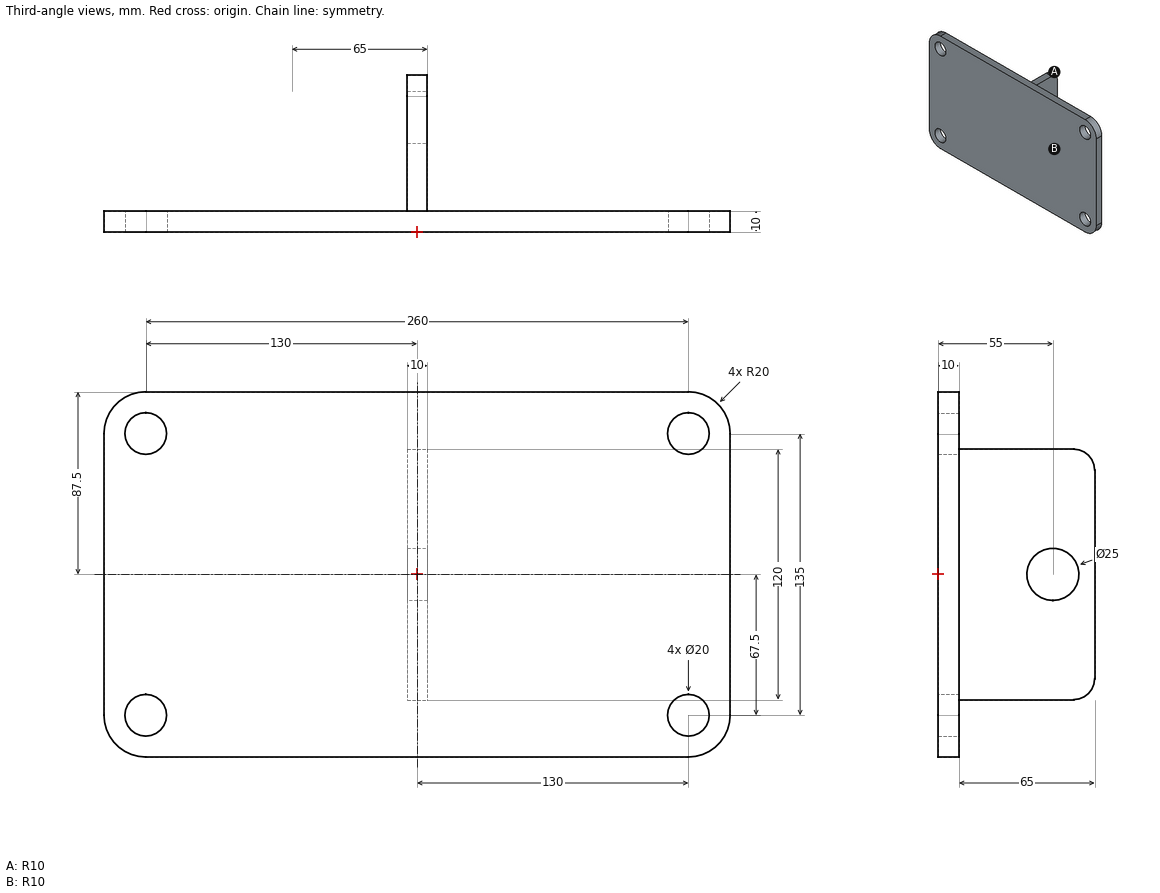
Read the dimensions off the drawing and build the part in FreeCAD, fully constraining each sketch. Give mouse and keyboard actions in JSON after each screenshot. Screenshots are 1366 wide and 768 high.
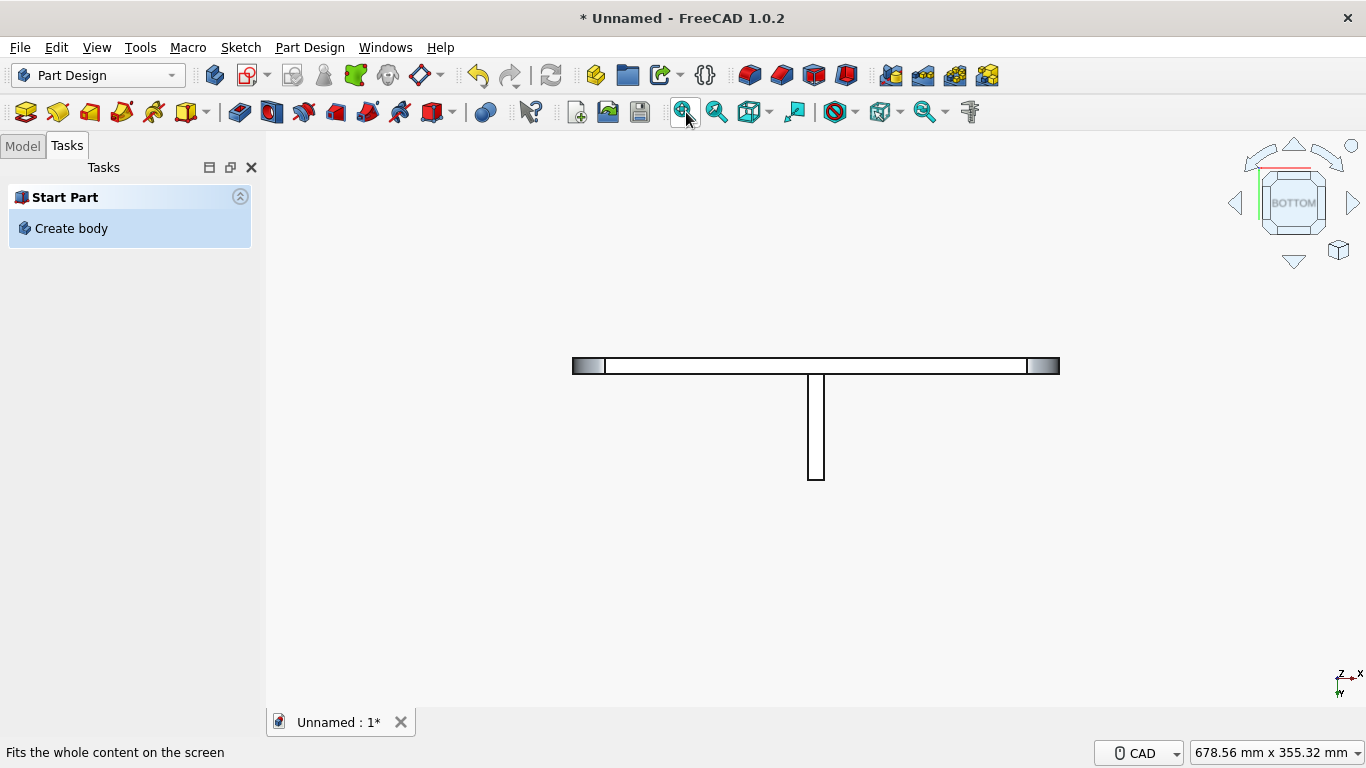
{"action": "left_click", "coordinate": [686, 112]}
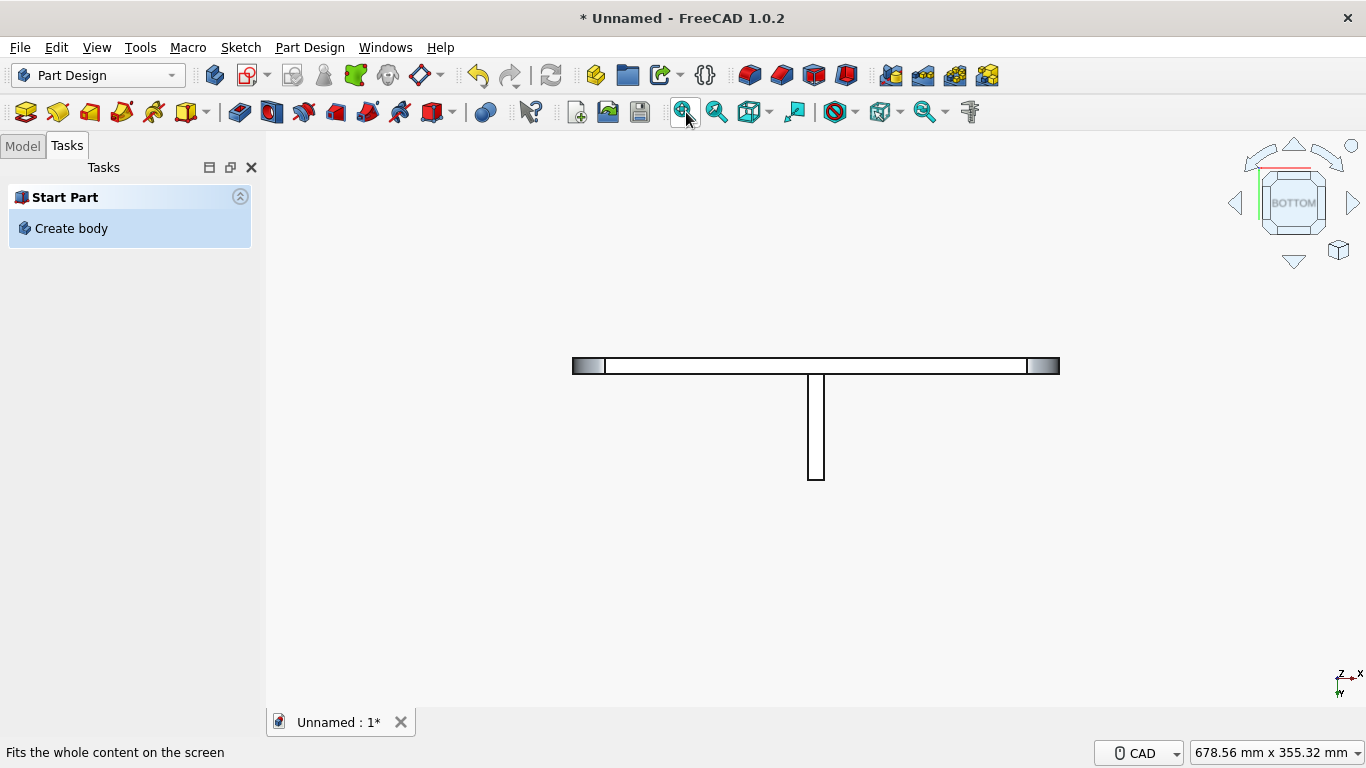
{"action": "scroll", "coordinate": [816, 479], "scroll_direction": "up", "scroll_amount": 5}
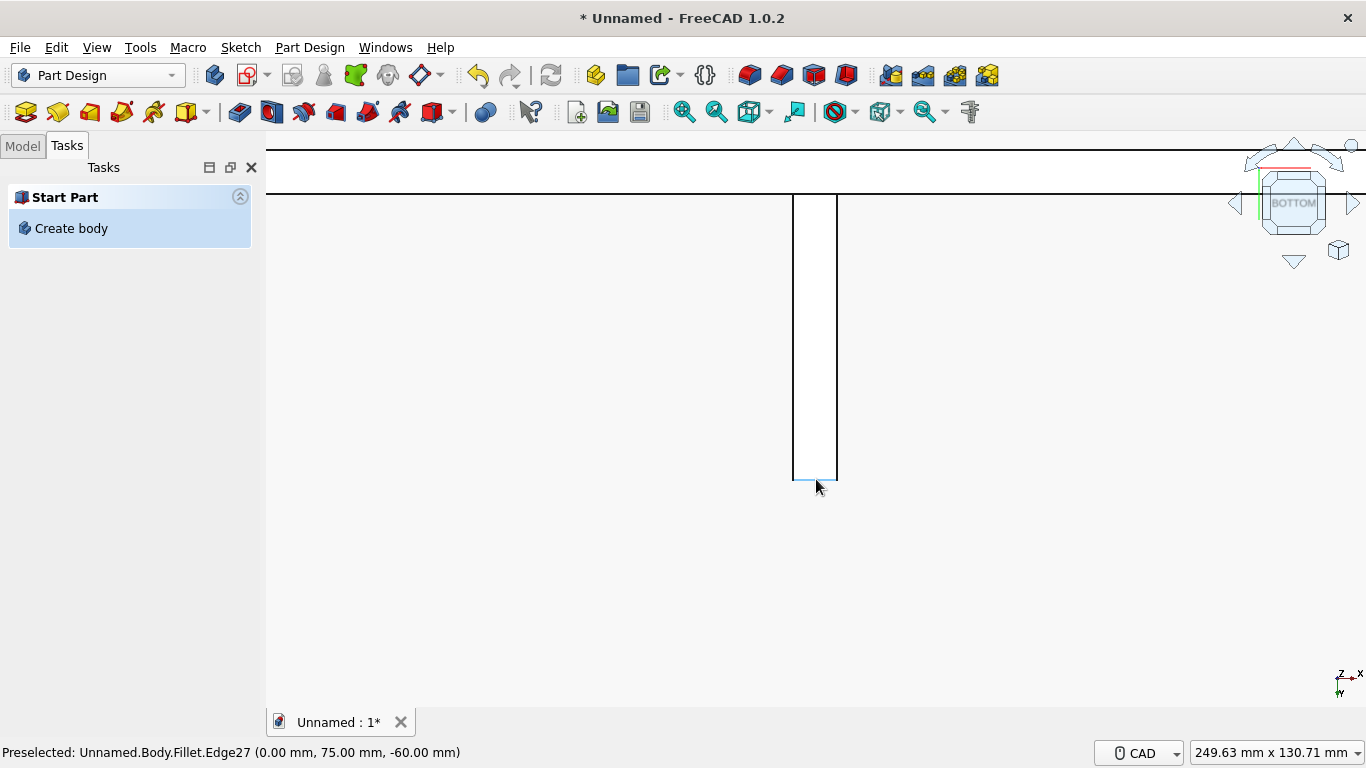
{"action": "left_click", "coordinate": [686, 112]}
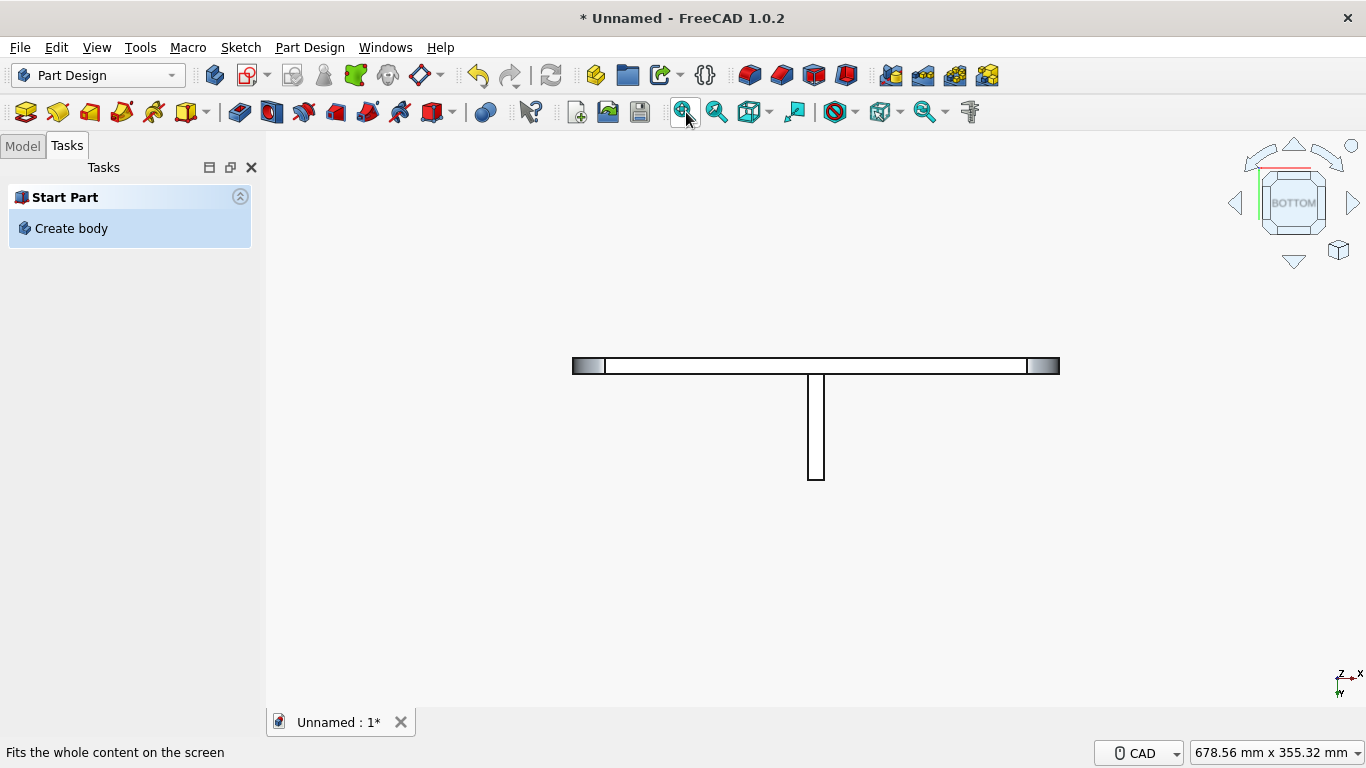
{"action": "key", "text": "4"}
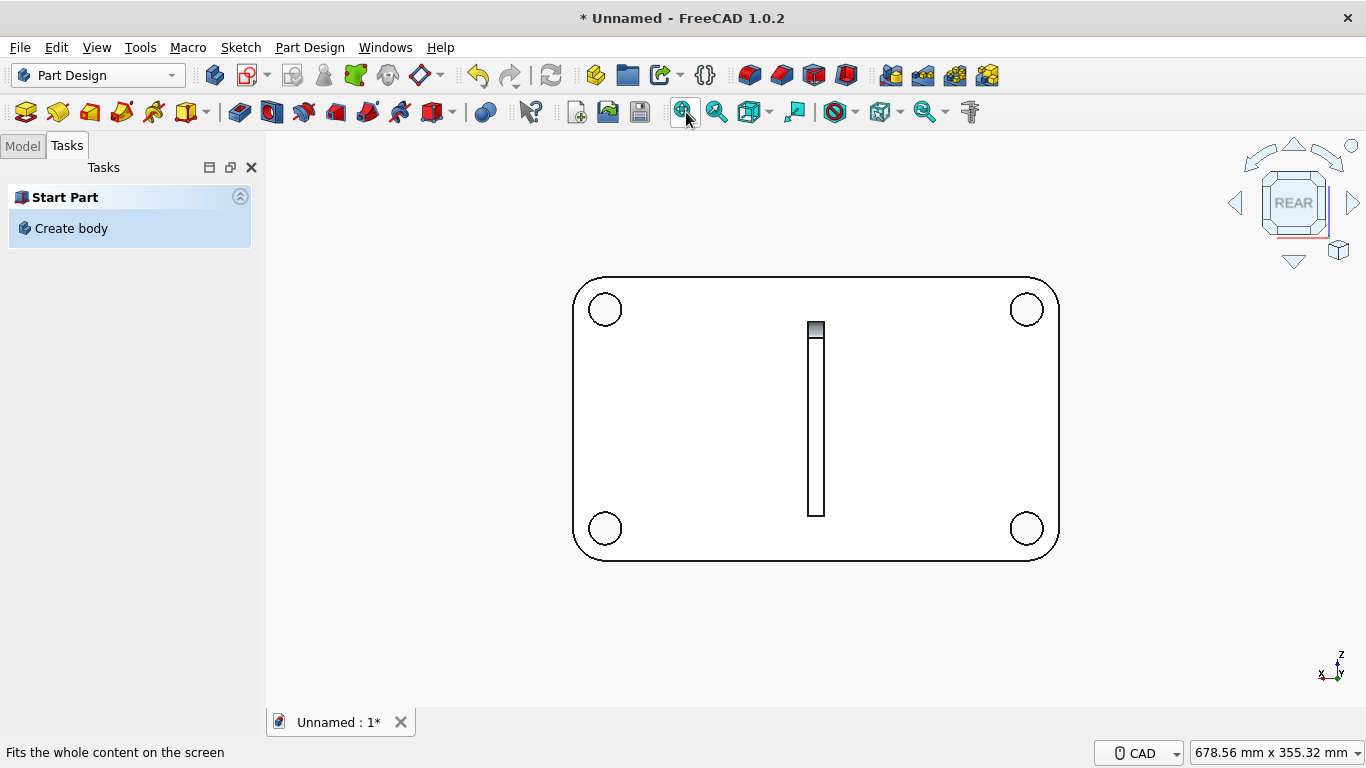
{"action": "left_click", "coordinate": [816, 515]}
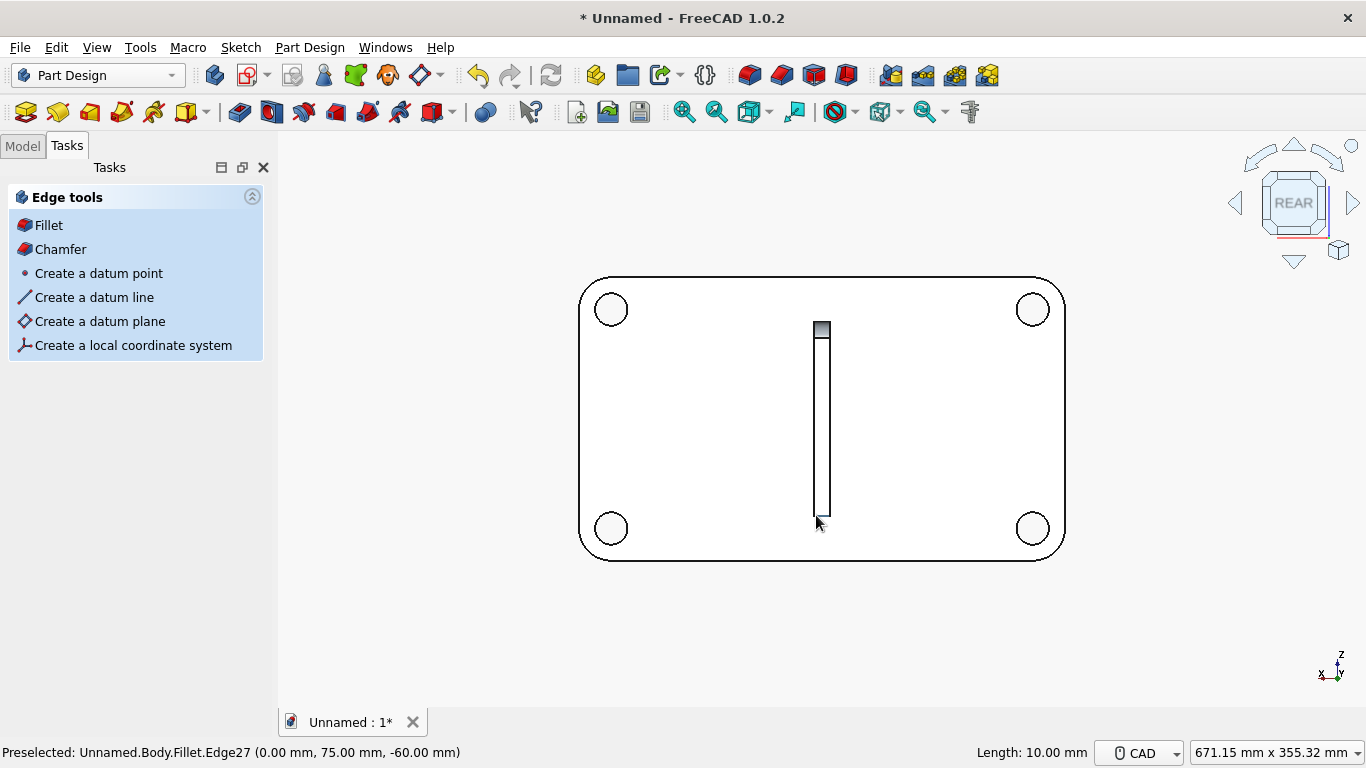
{"action": "left_click", "coordinate": [750, 76]}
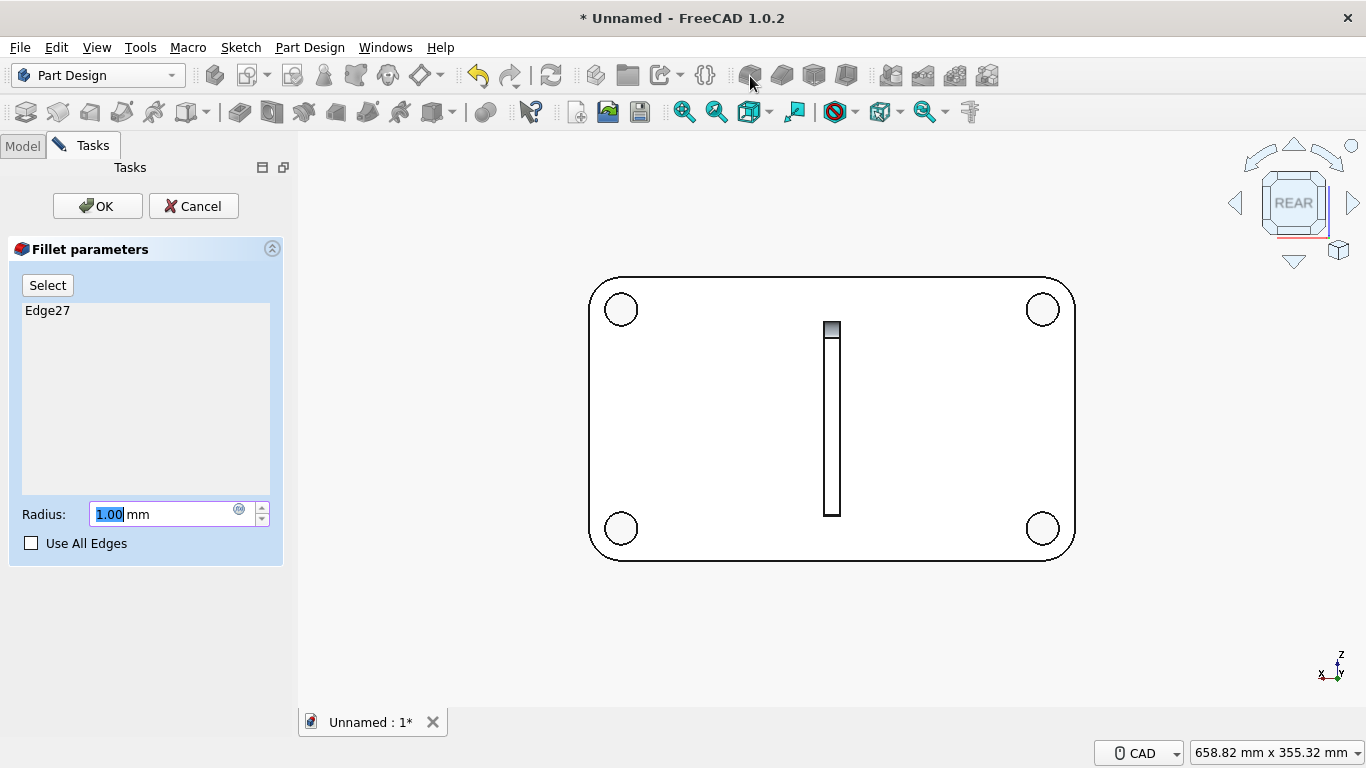
{"action": "type", "text": "10"}
{"action": "key", "text": "Tab"}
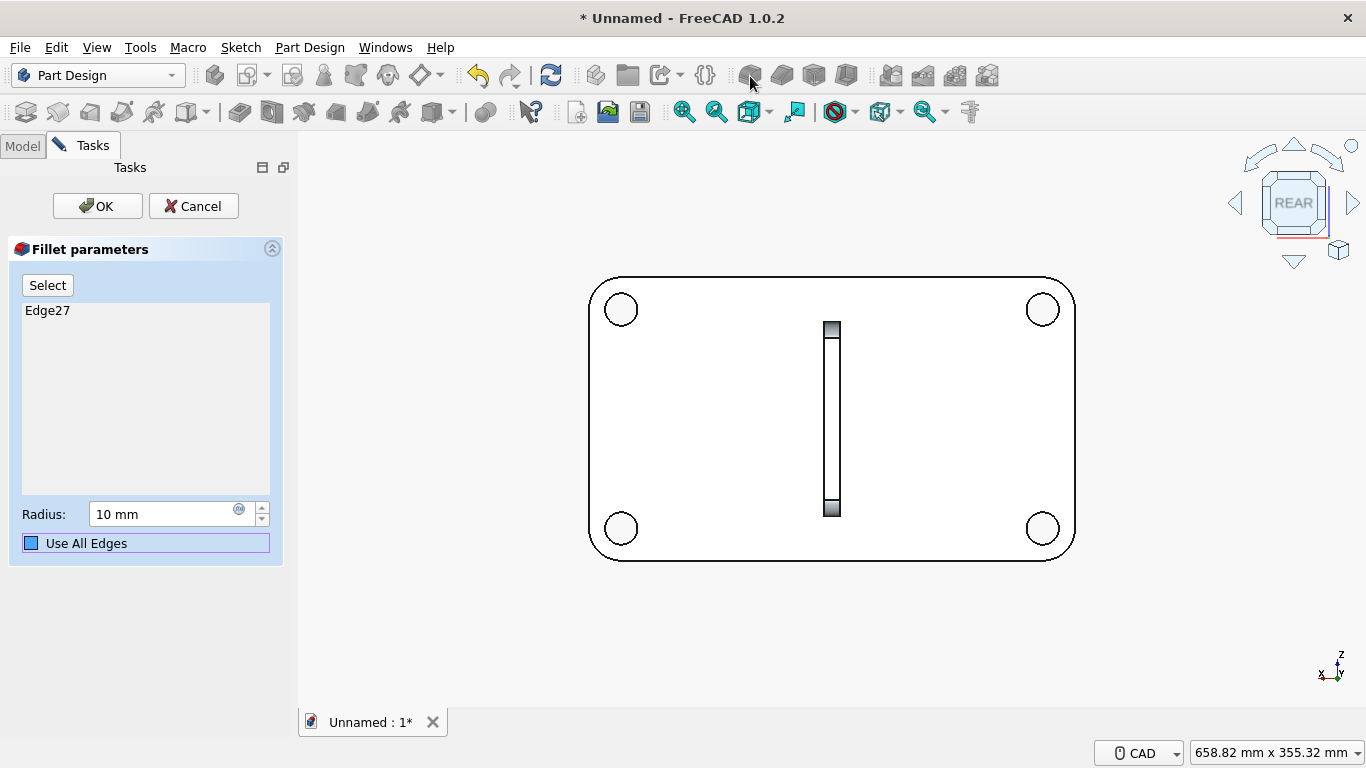
{"action": "left_click", "coordinate": [98, 206]}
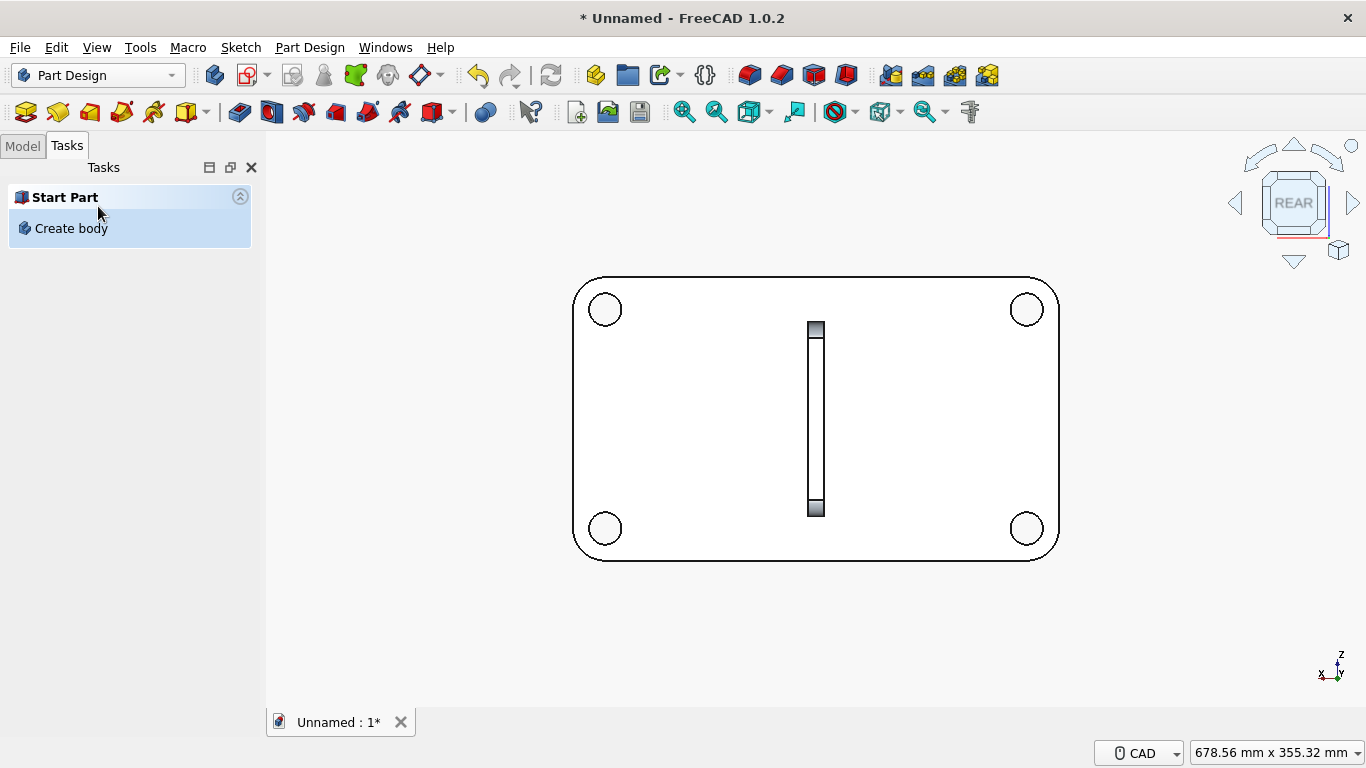
{"action": "key", "text": "0"}